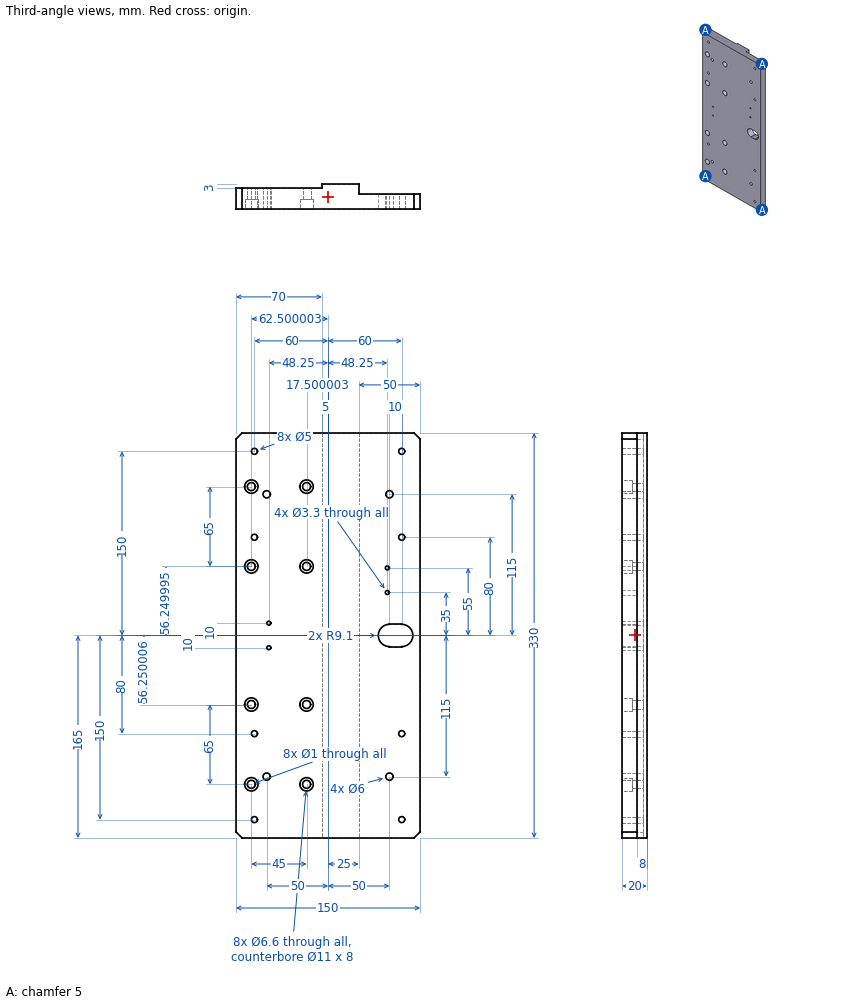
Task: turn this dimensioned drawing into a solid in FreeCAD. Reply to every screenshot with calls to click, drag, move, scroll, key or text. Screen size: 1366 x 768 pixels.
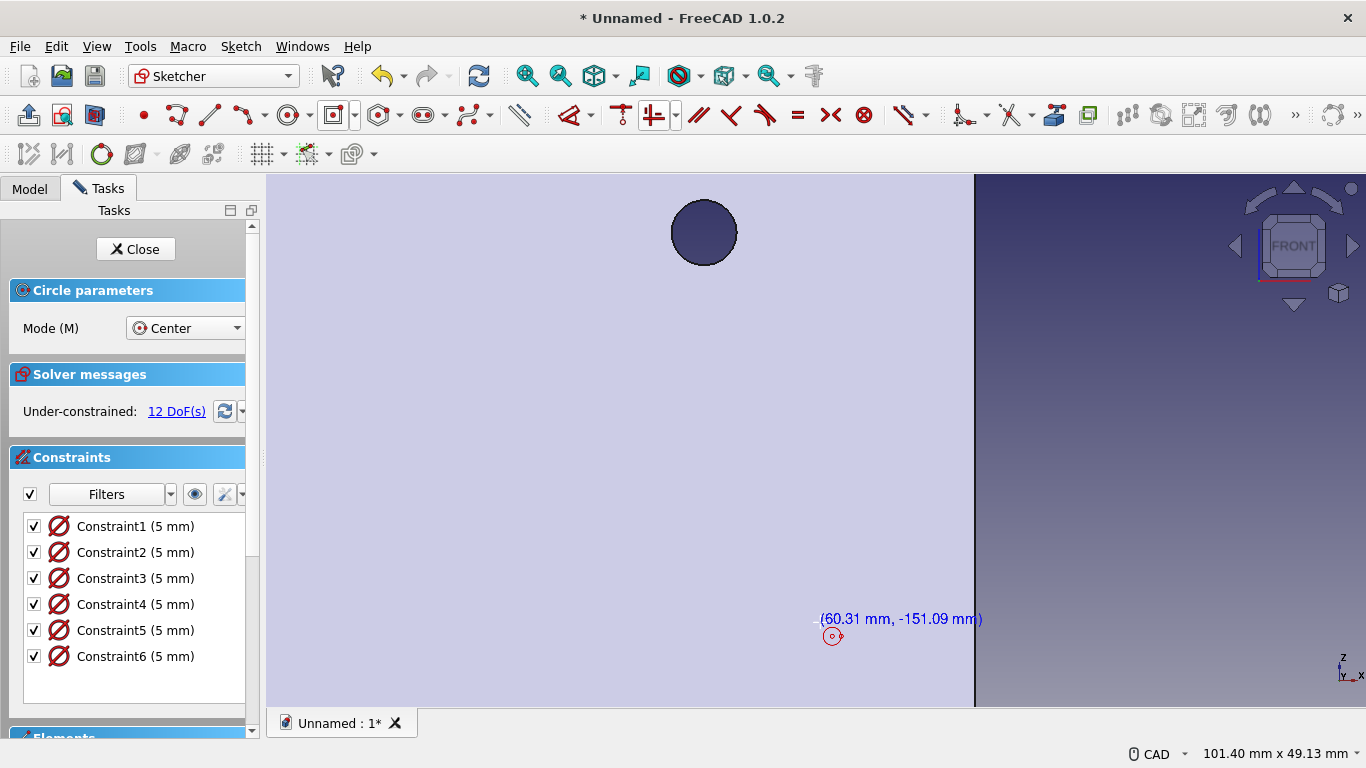
scroll(820, 622, down, 11)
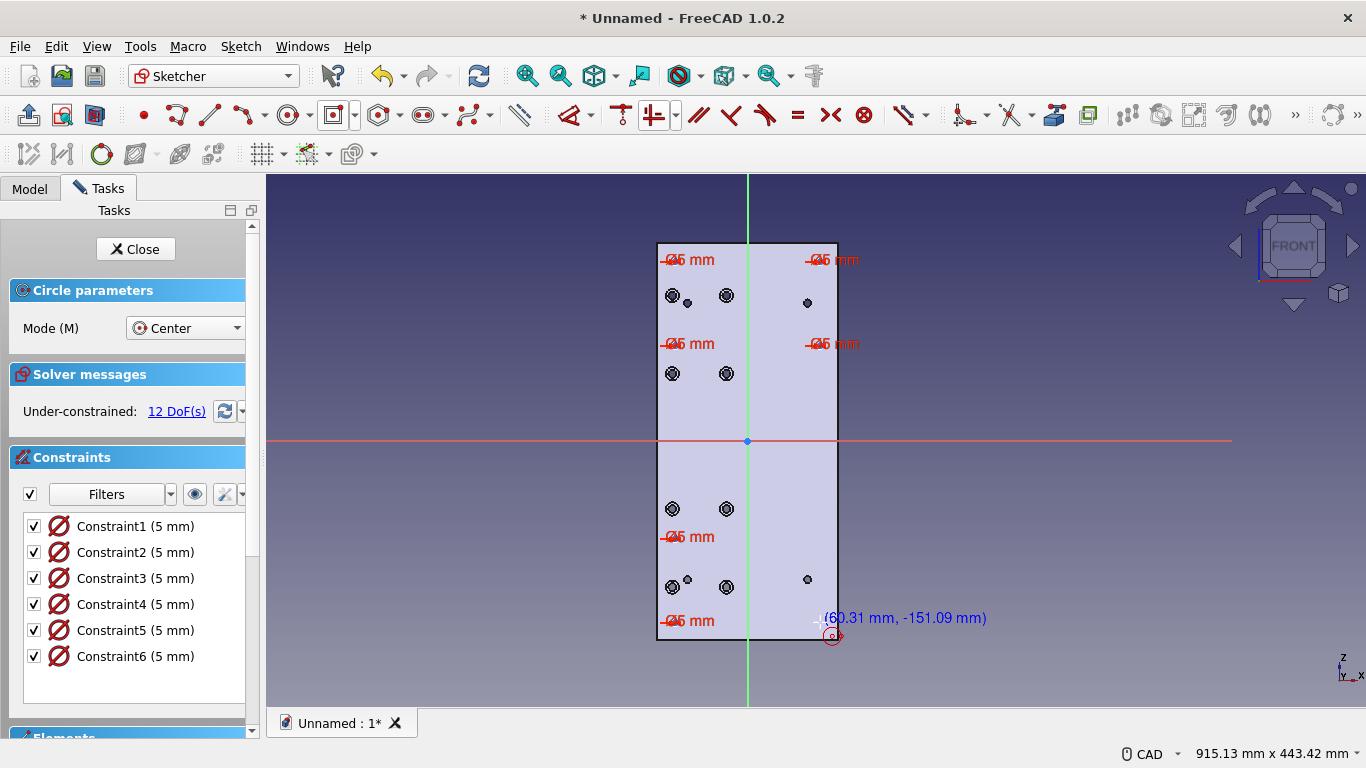
click(820, 622)
move(822, 620)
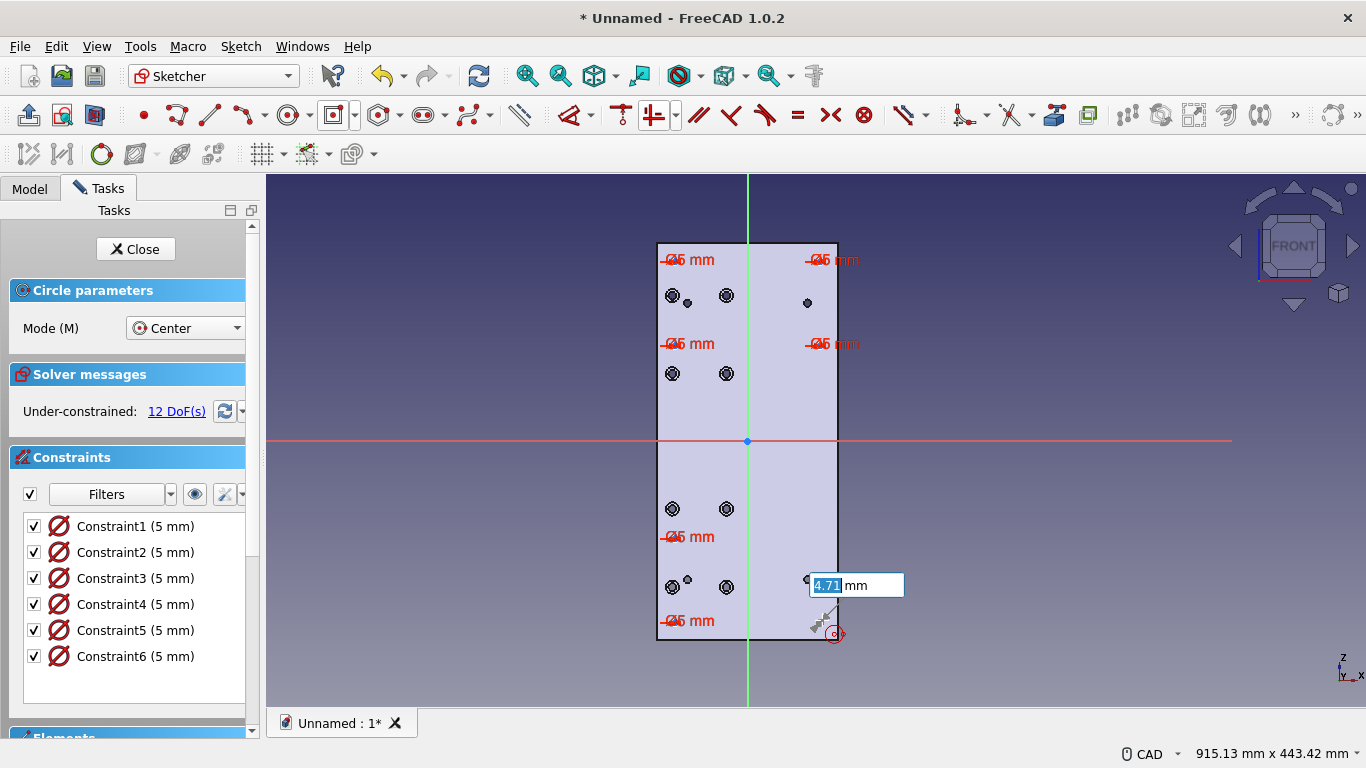
text(5)
key(Return)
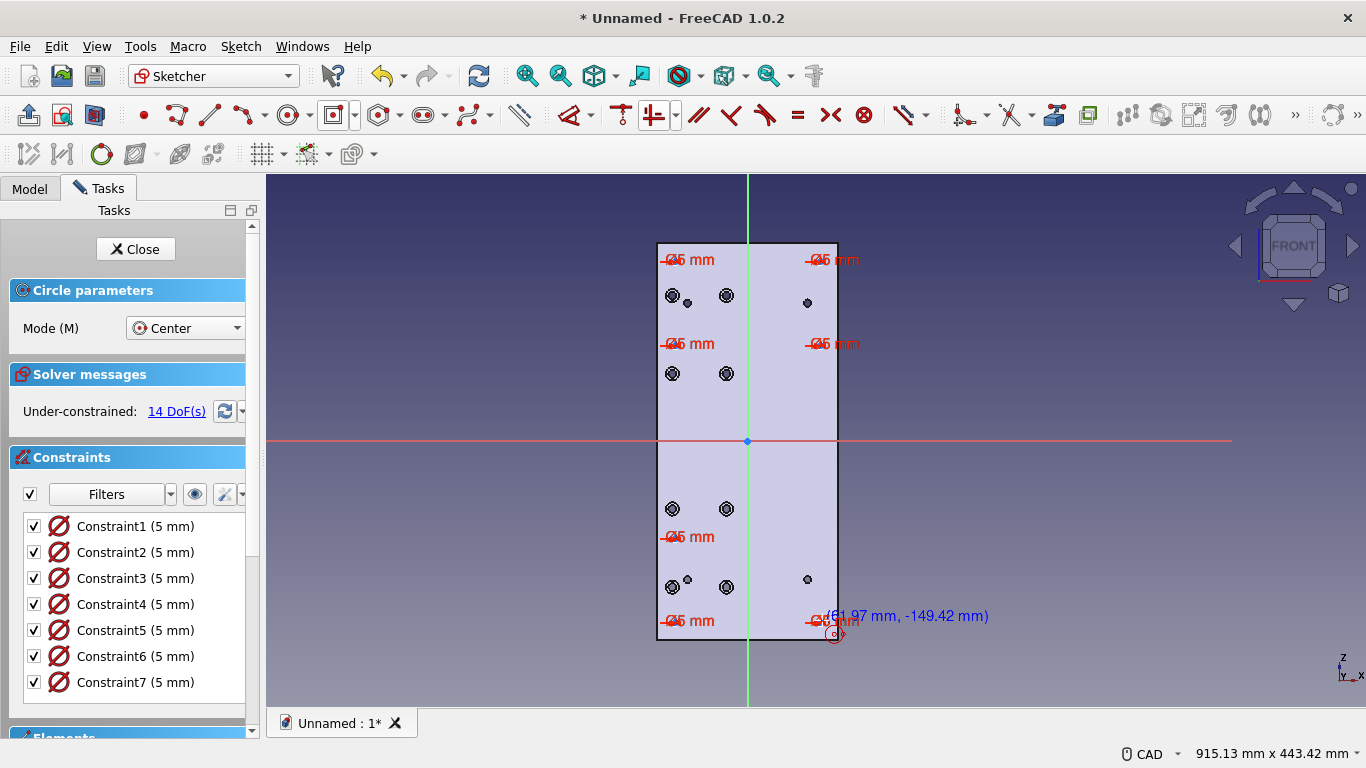
scroll(820, 538, up, 11)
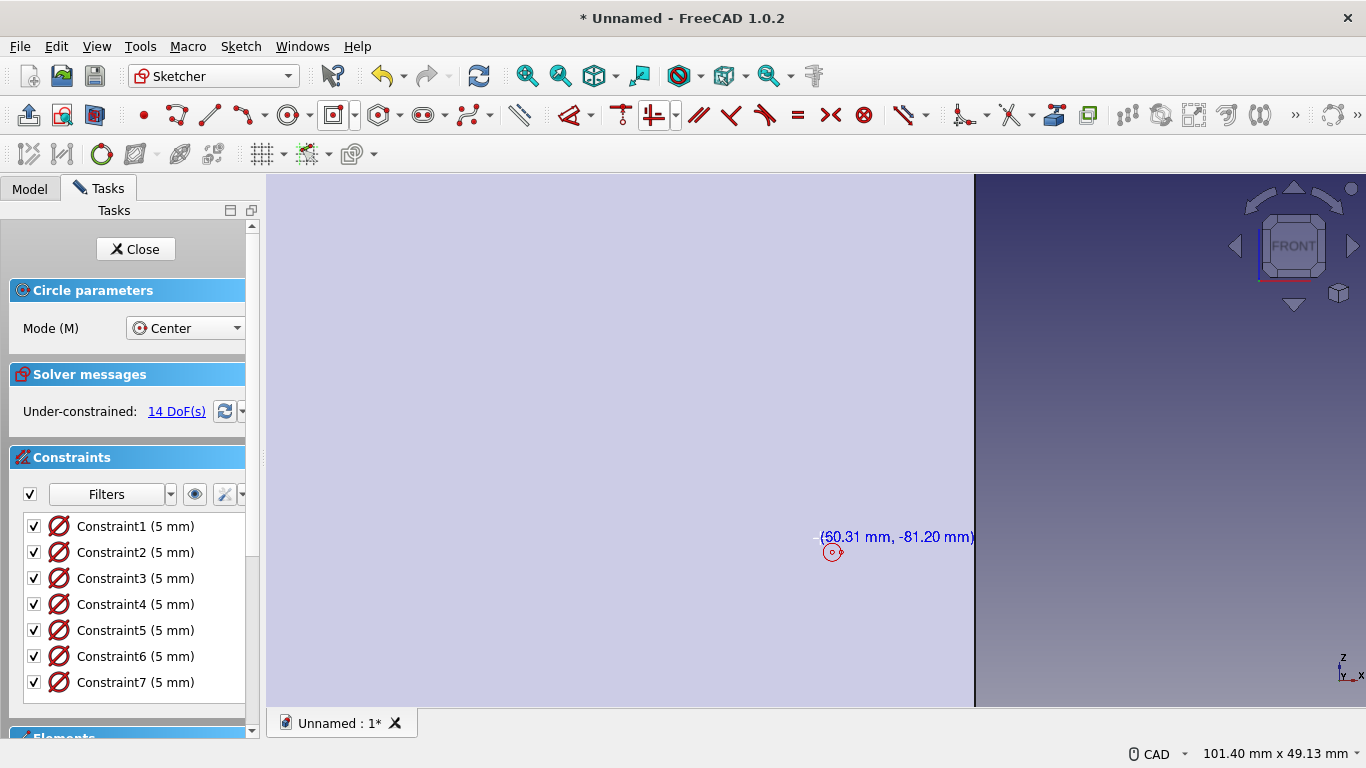
scroll(820, 538, down, 11)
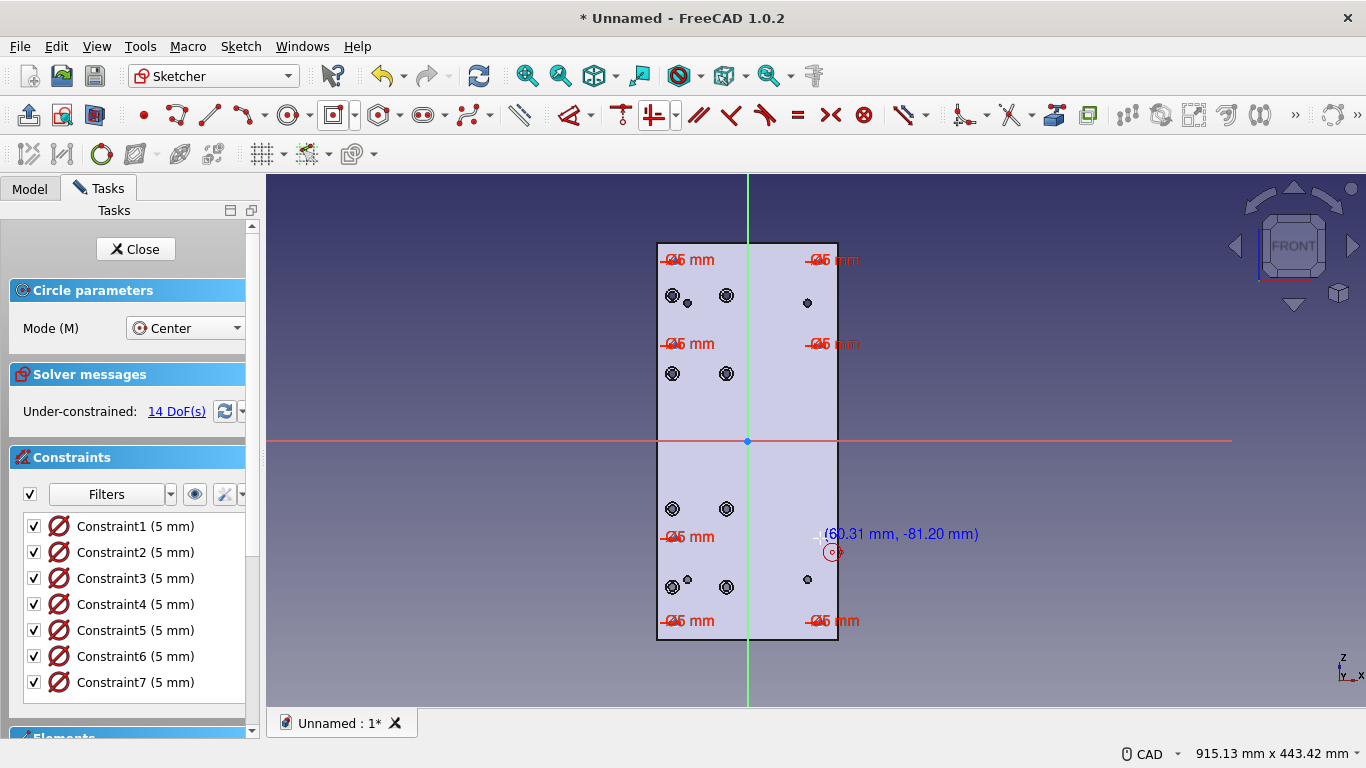
click(820, 538)
move(822, 535)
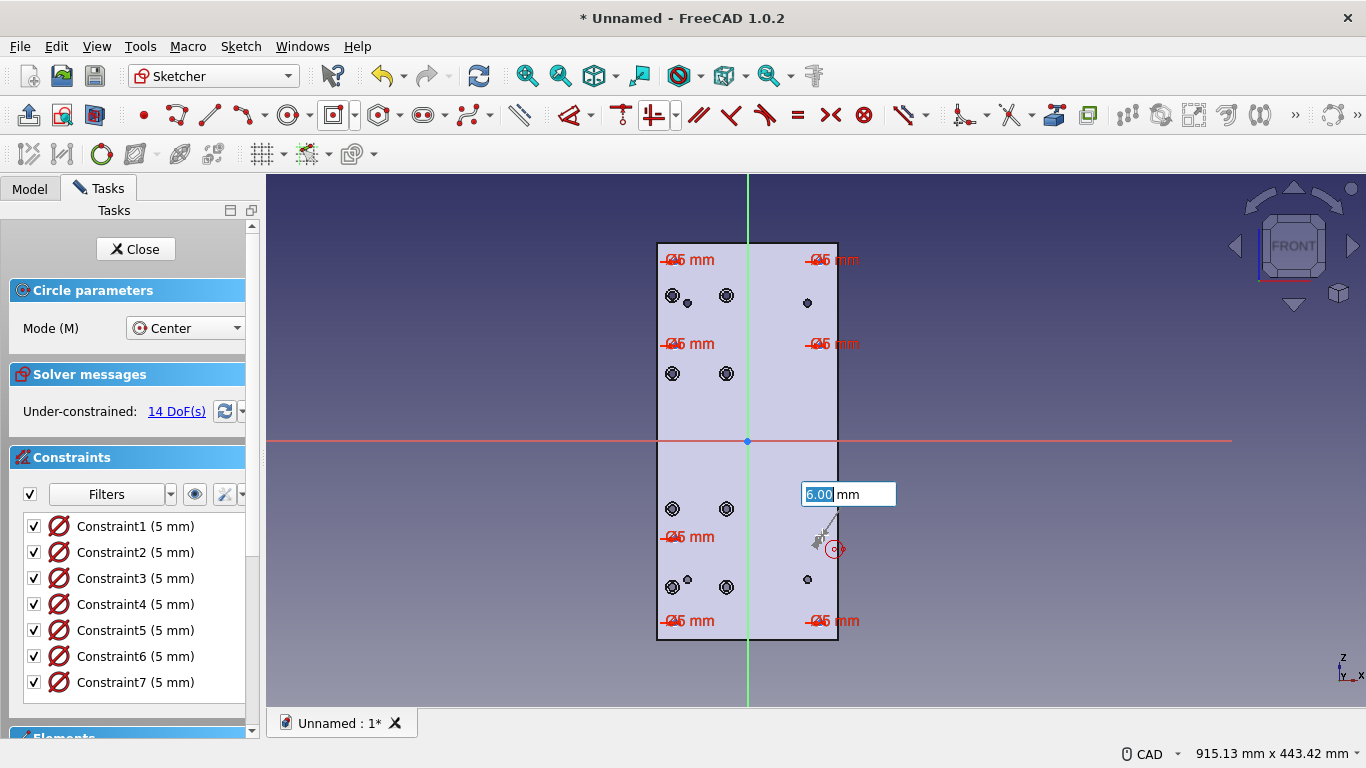
text(5)
key(Return)
key(Escape)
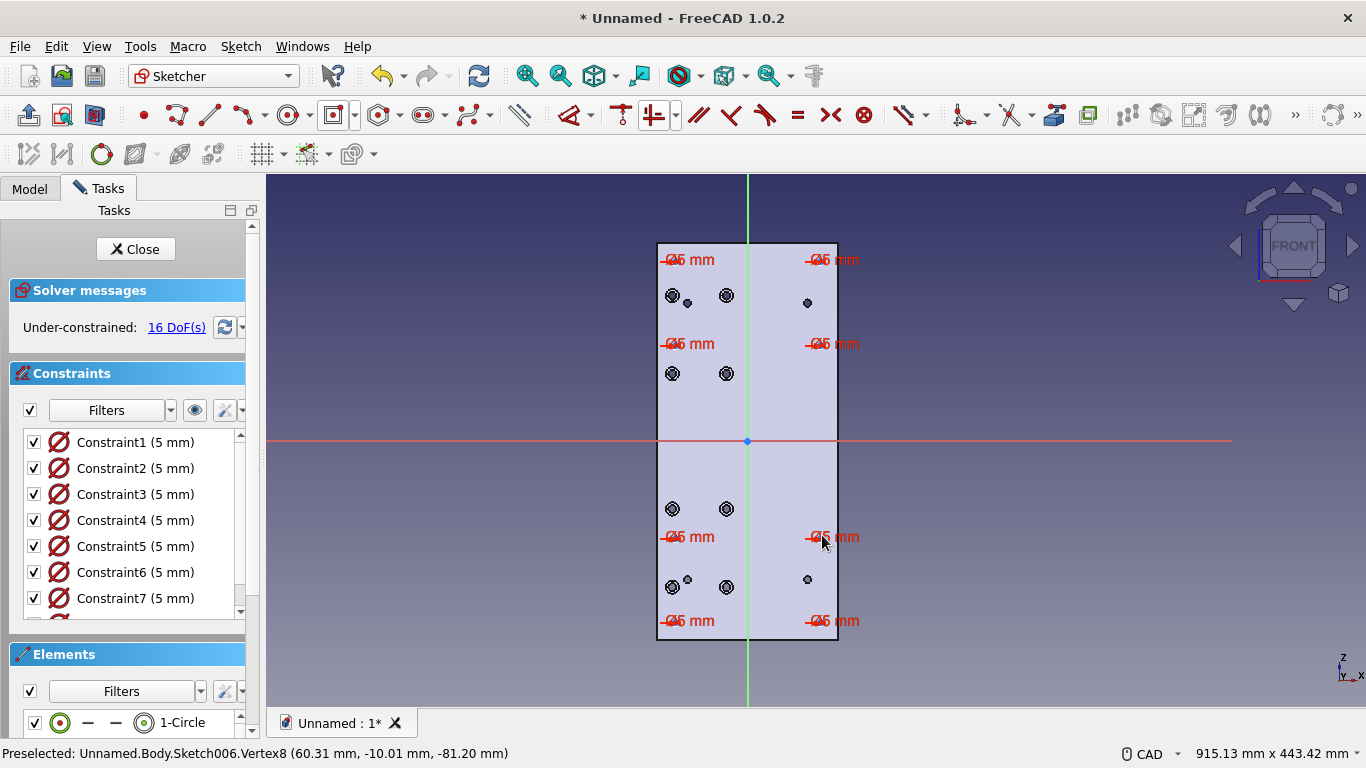
click(675, 262)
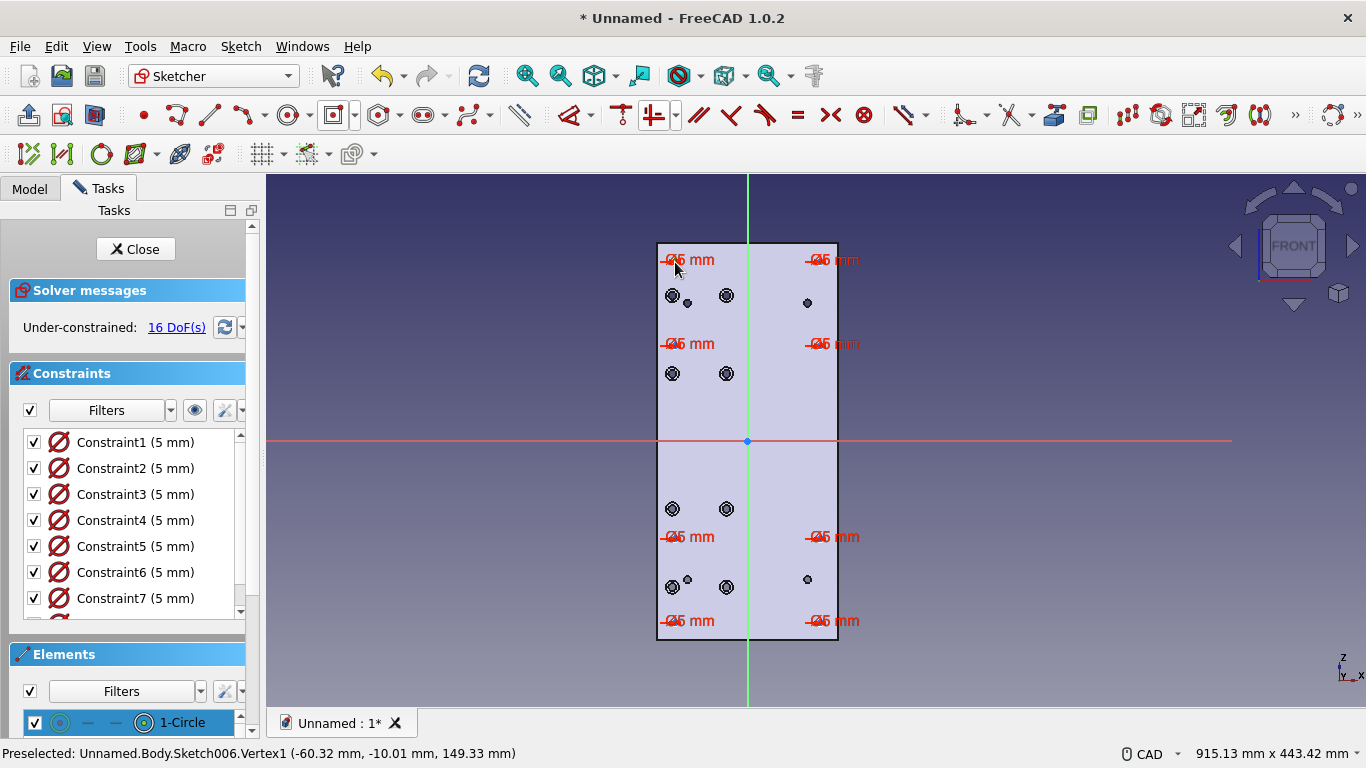
click(820, 262)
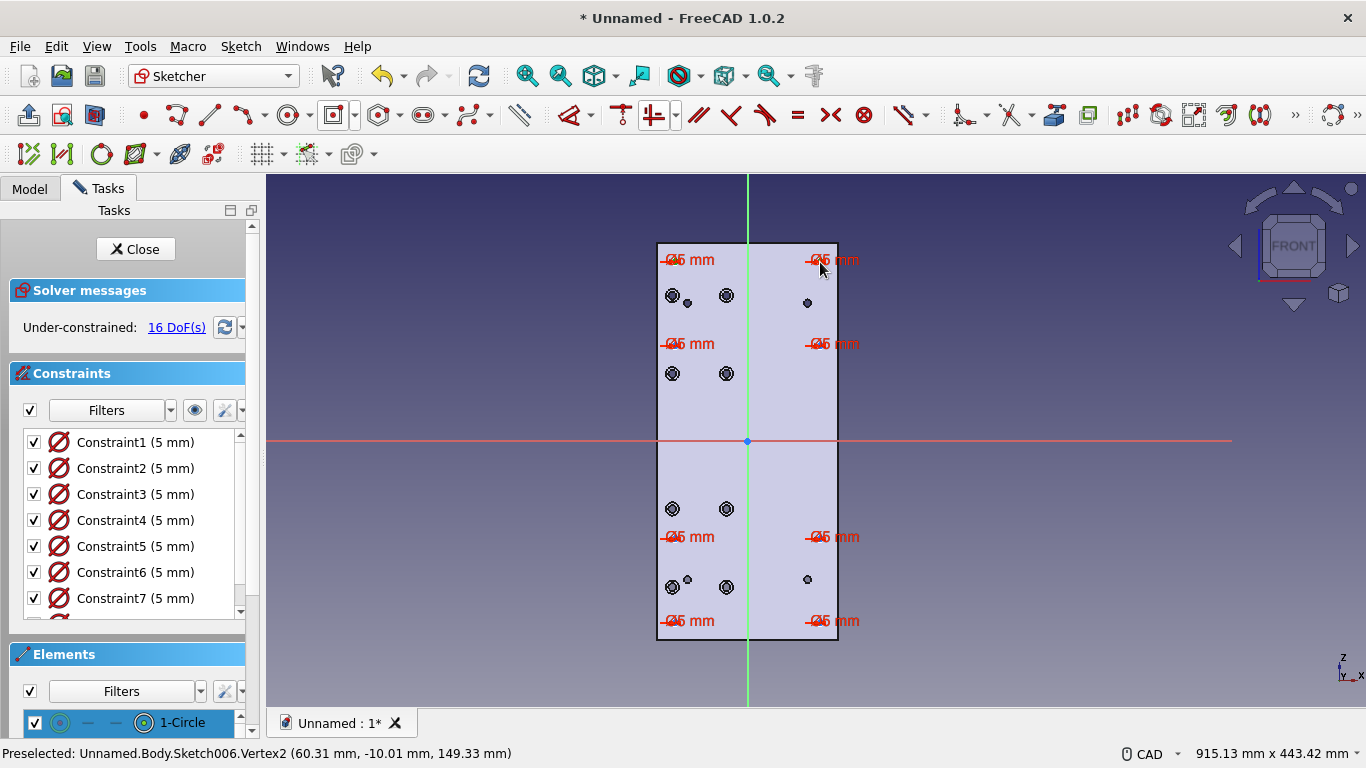
key(h)